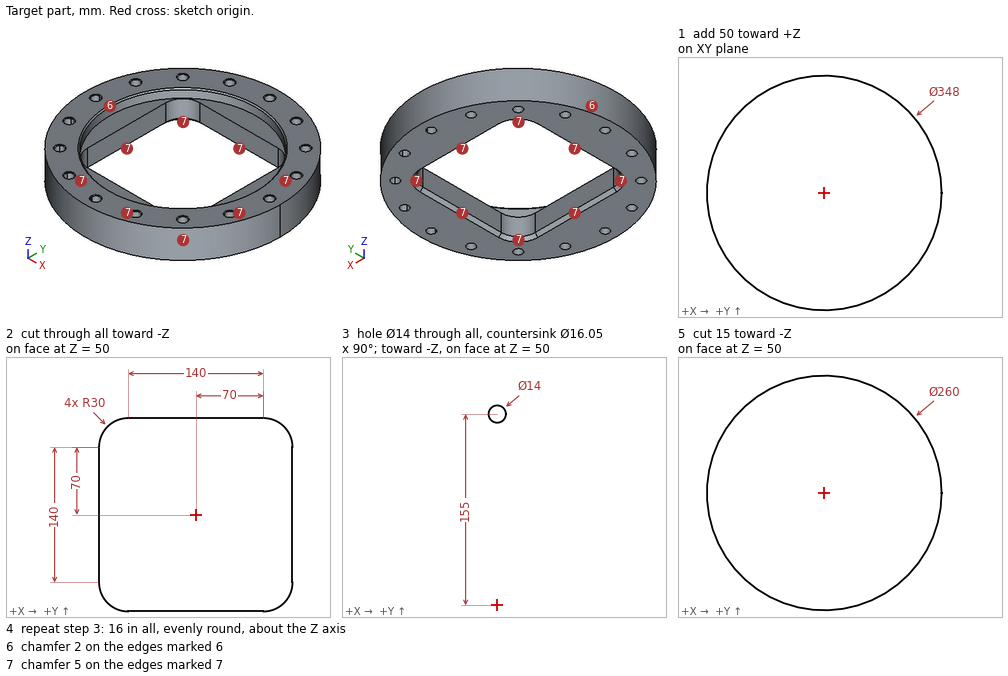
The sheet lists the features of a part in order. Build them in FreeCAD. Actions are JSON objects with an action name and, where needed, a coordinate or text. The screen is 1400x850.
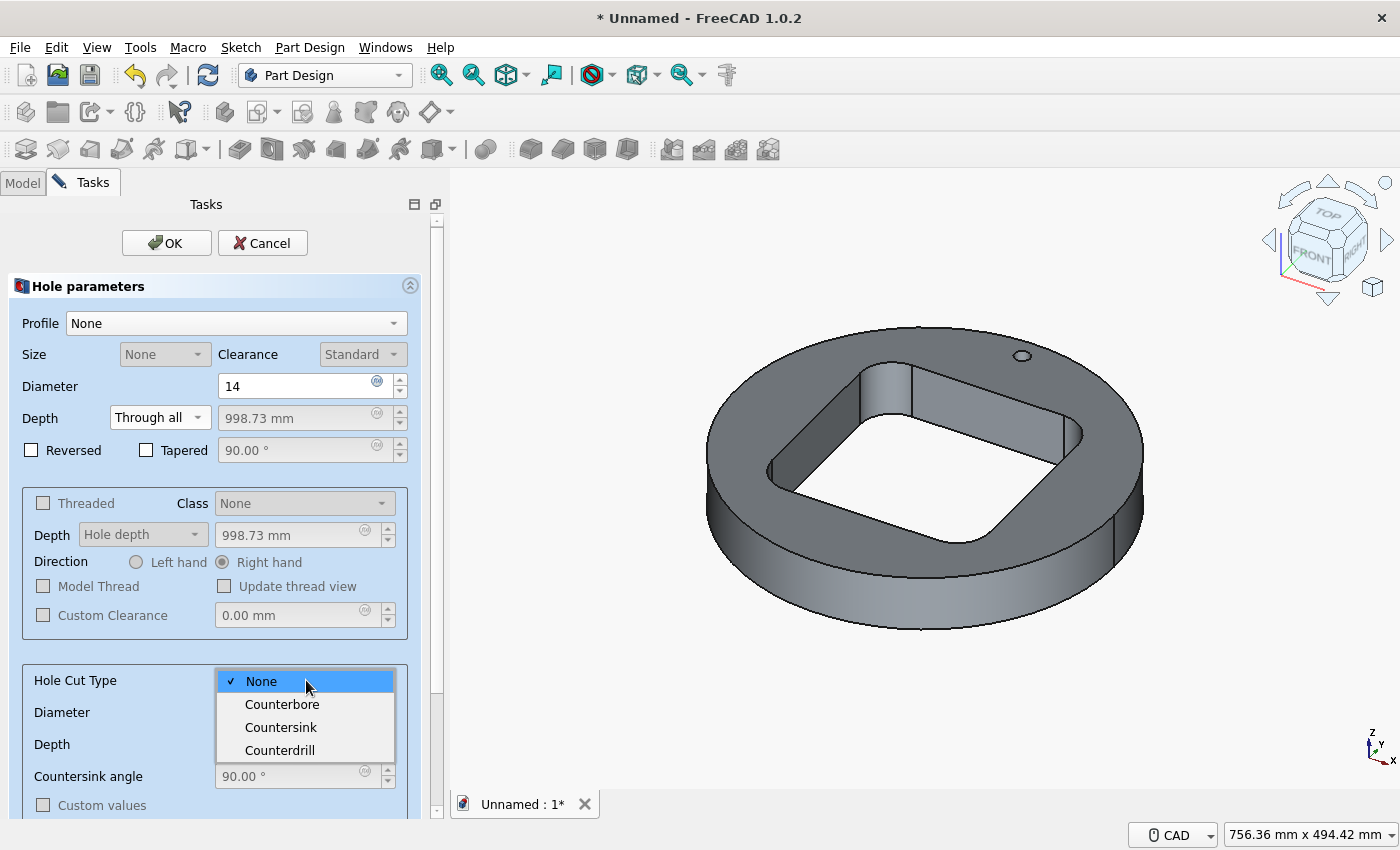
{"action": "left_click", "coordinate": [304, 728]}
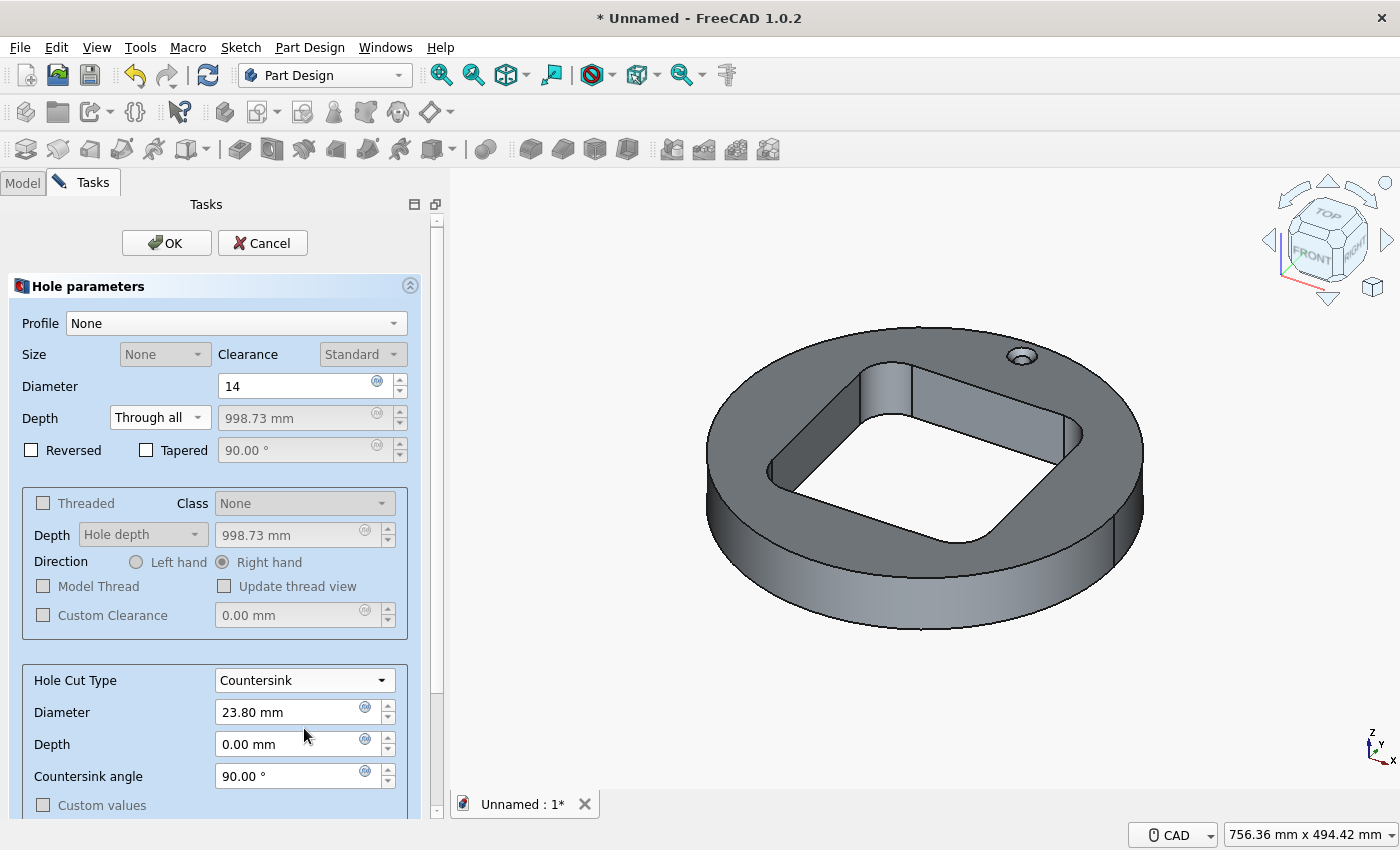
{"action": "triple_click", "coordinate": [298, 712]}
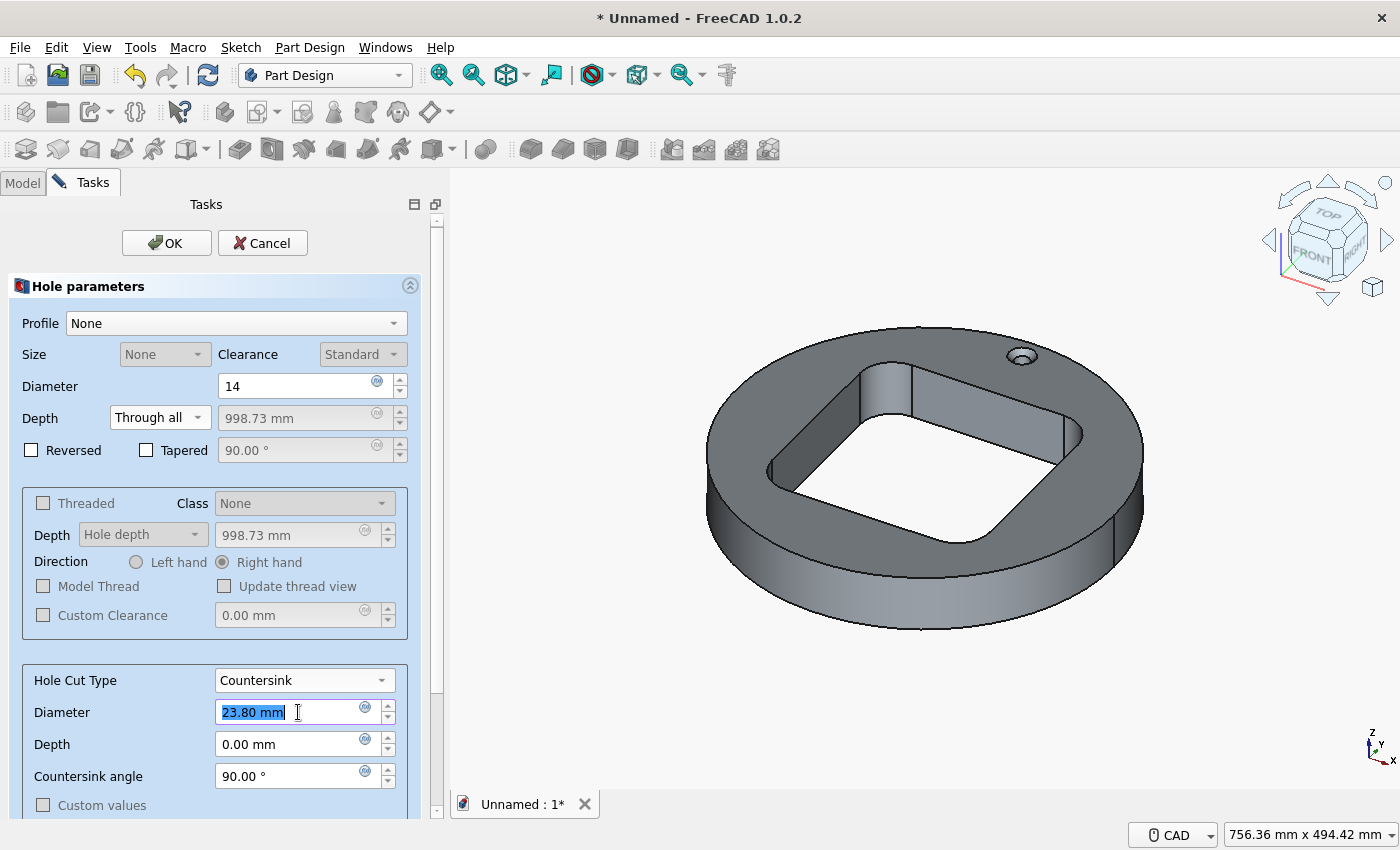
{"action": "type", "text": "16.05"}
{"action": "key", "text": "Tab"}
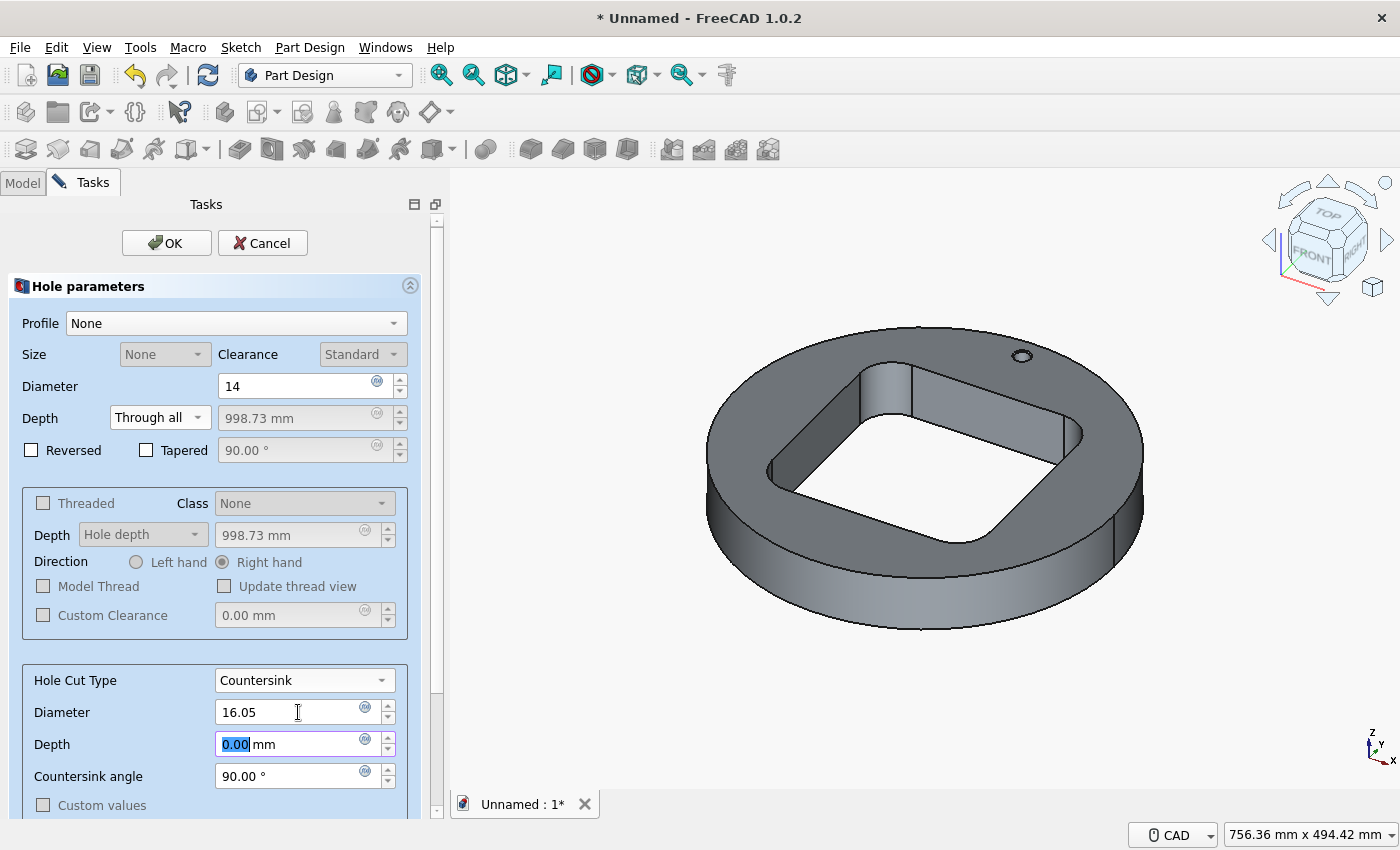
{"action": "left_click", "coordinate": [167, 243]}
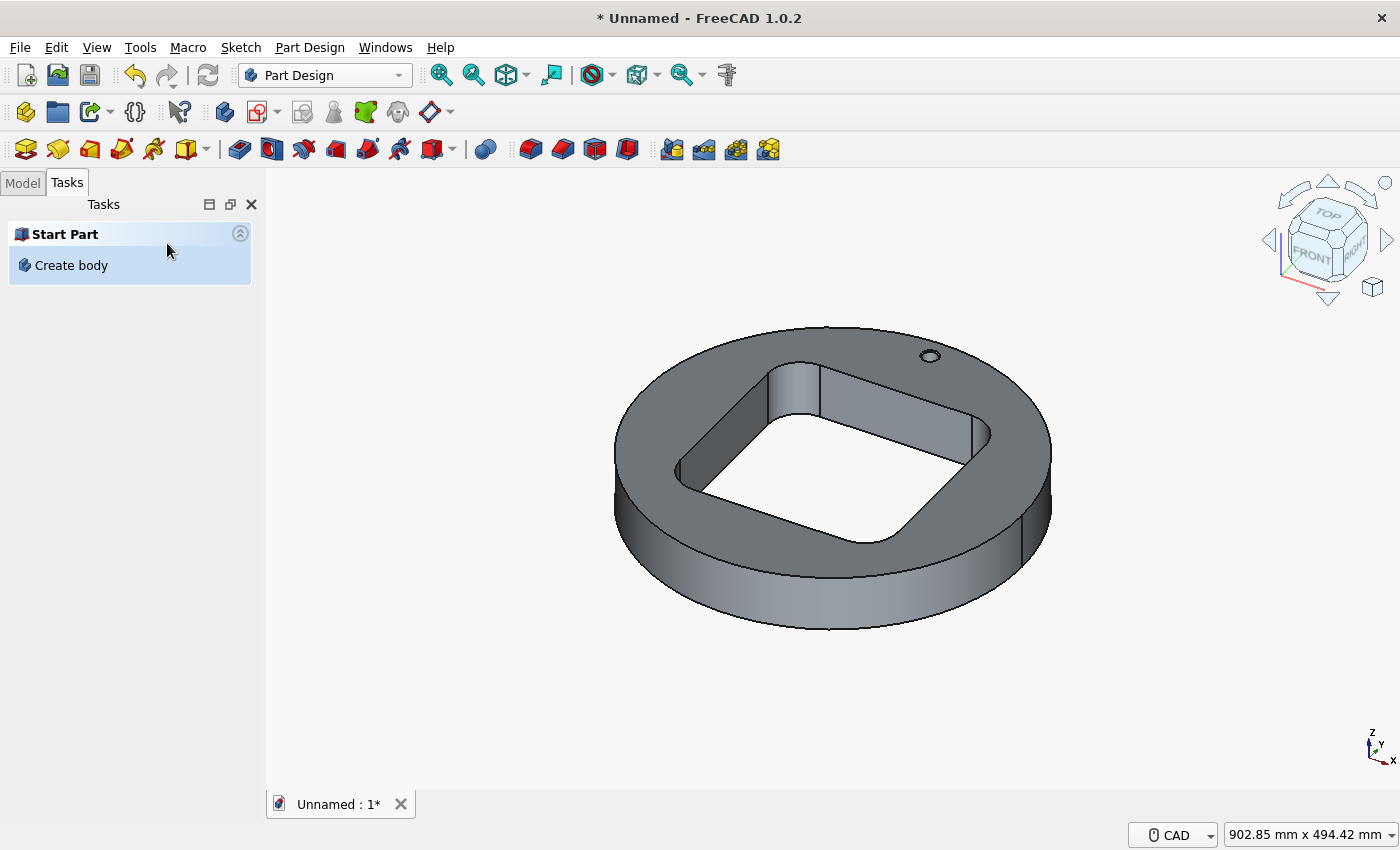
{"action": "left_click", "coordinate": [23, 182]}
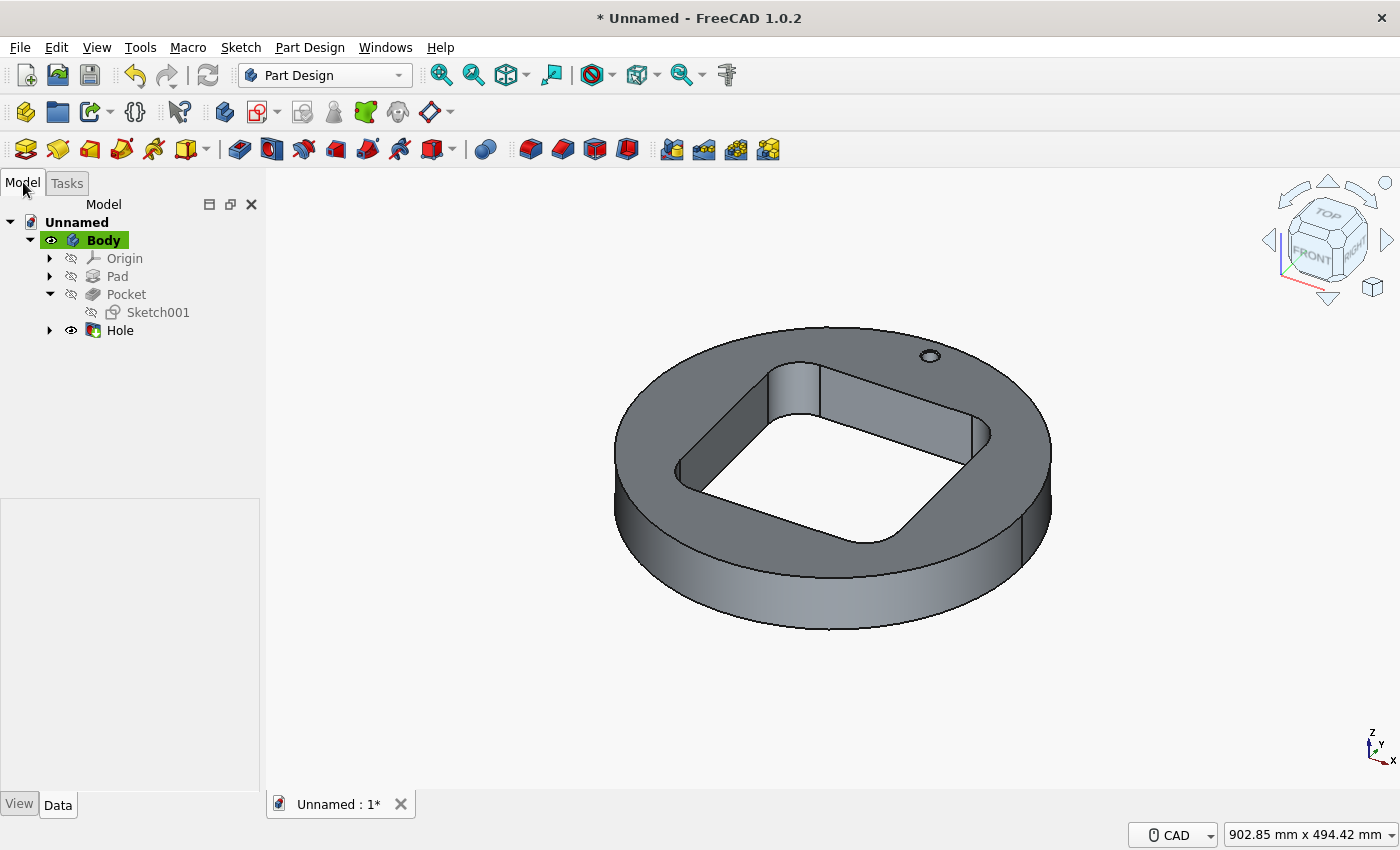
{"action": "left_click", "coordinate": [116, 330]}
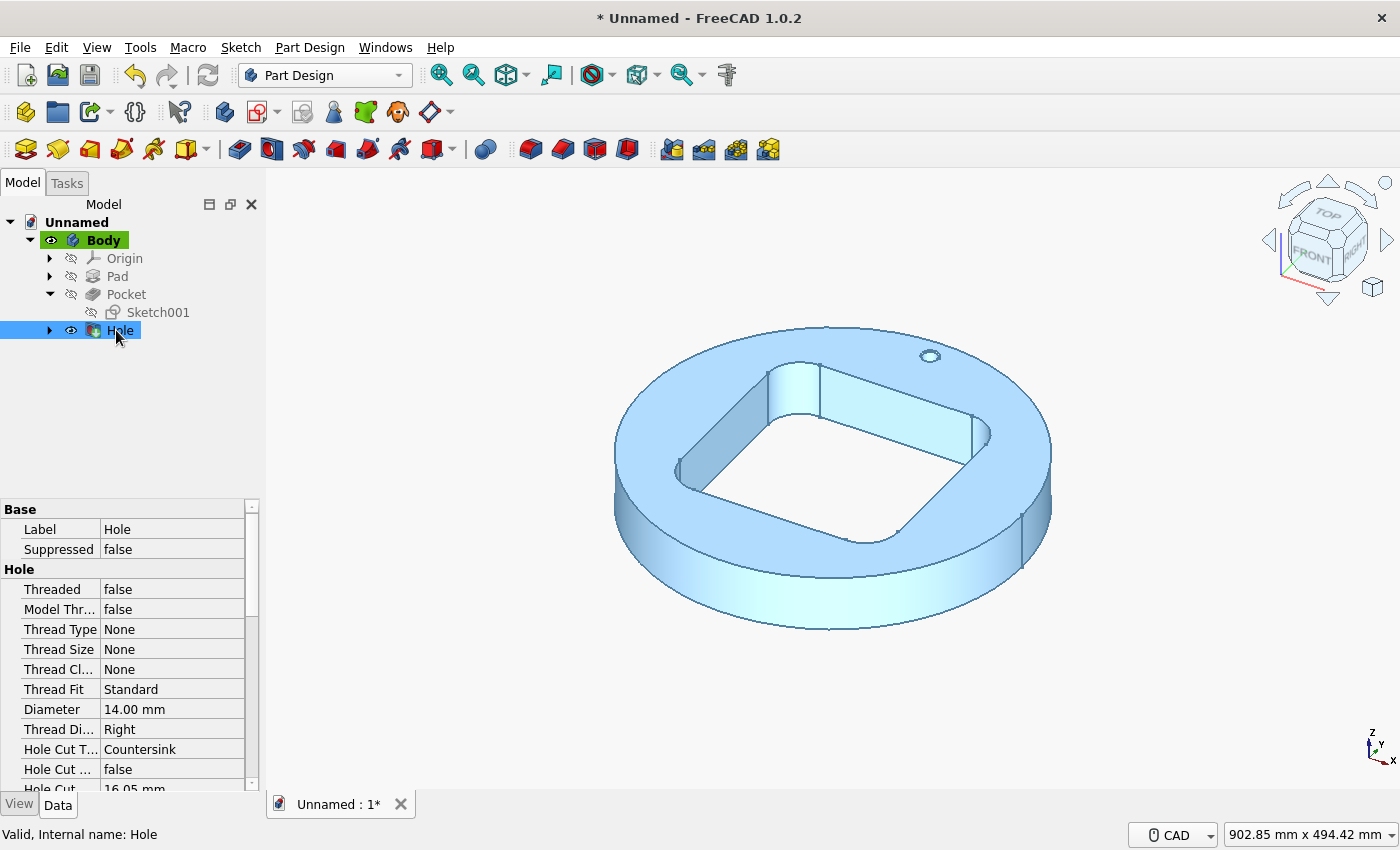
{"action": "left_click", "coordinate": [736, 150]}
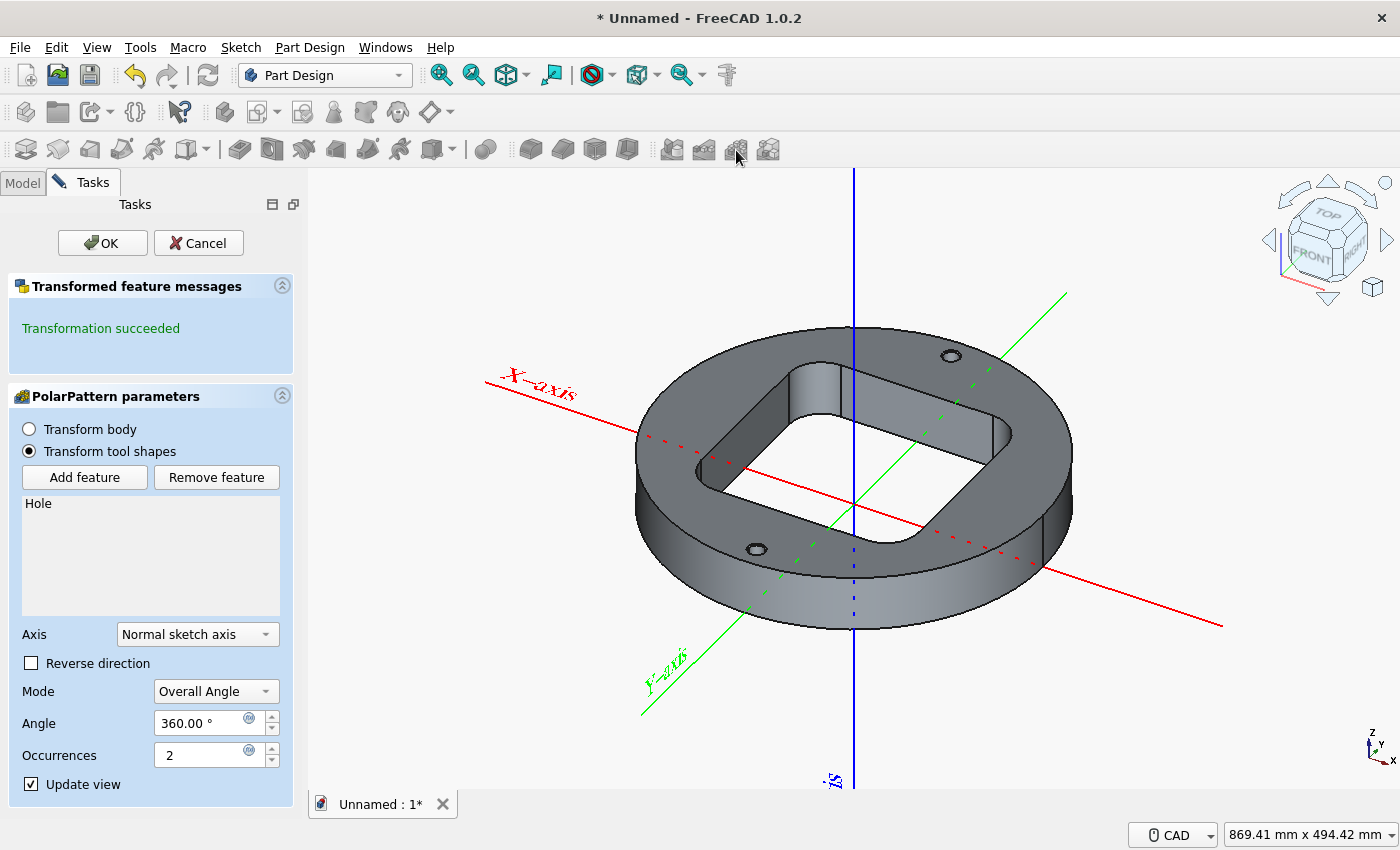
{"action": "left_click", "coordinate": [198, 634]}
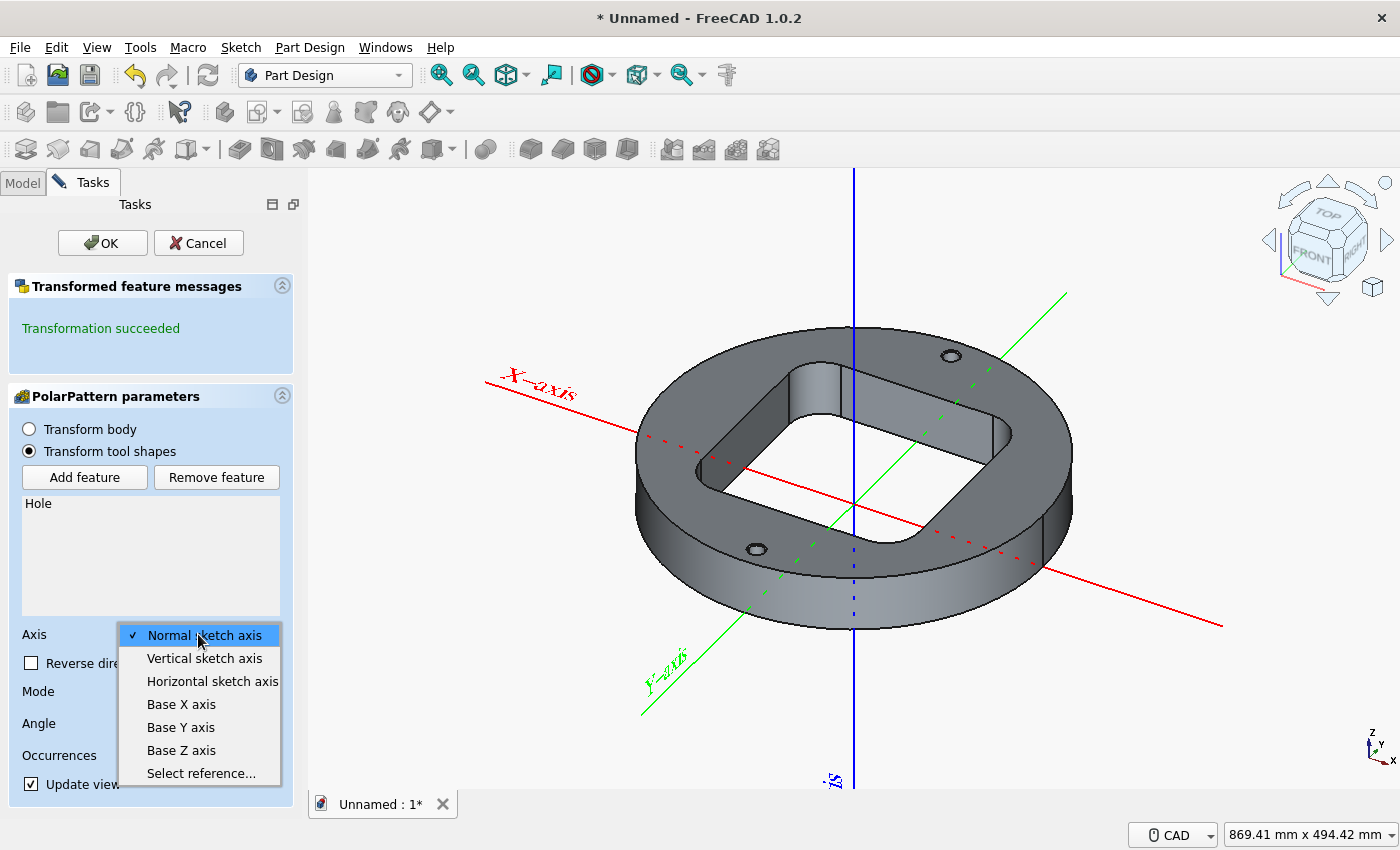
{"action": "left_click", "coordinate": [198, 750]}